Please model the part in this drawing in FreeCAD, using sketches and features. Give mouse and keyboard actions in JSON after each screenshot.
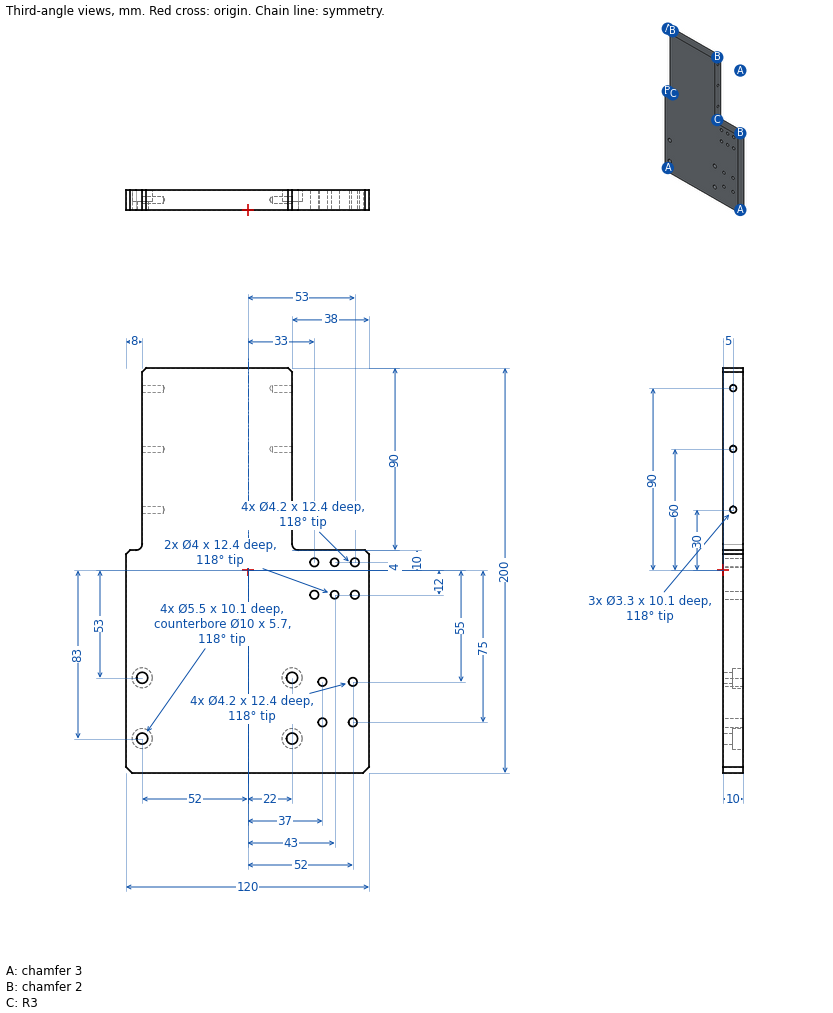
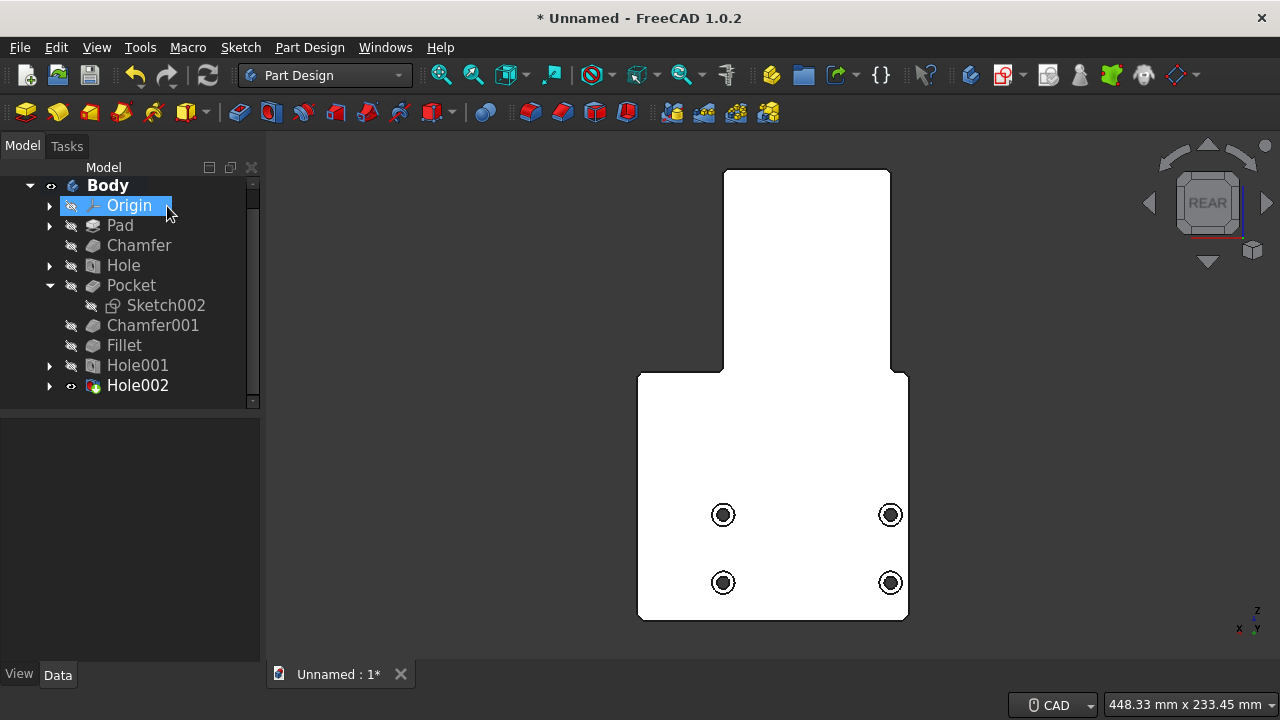
{"action": "left_click", "coordinate": [812, 459]}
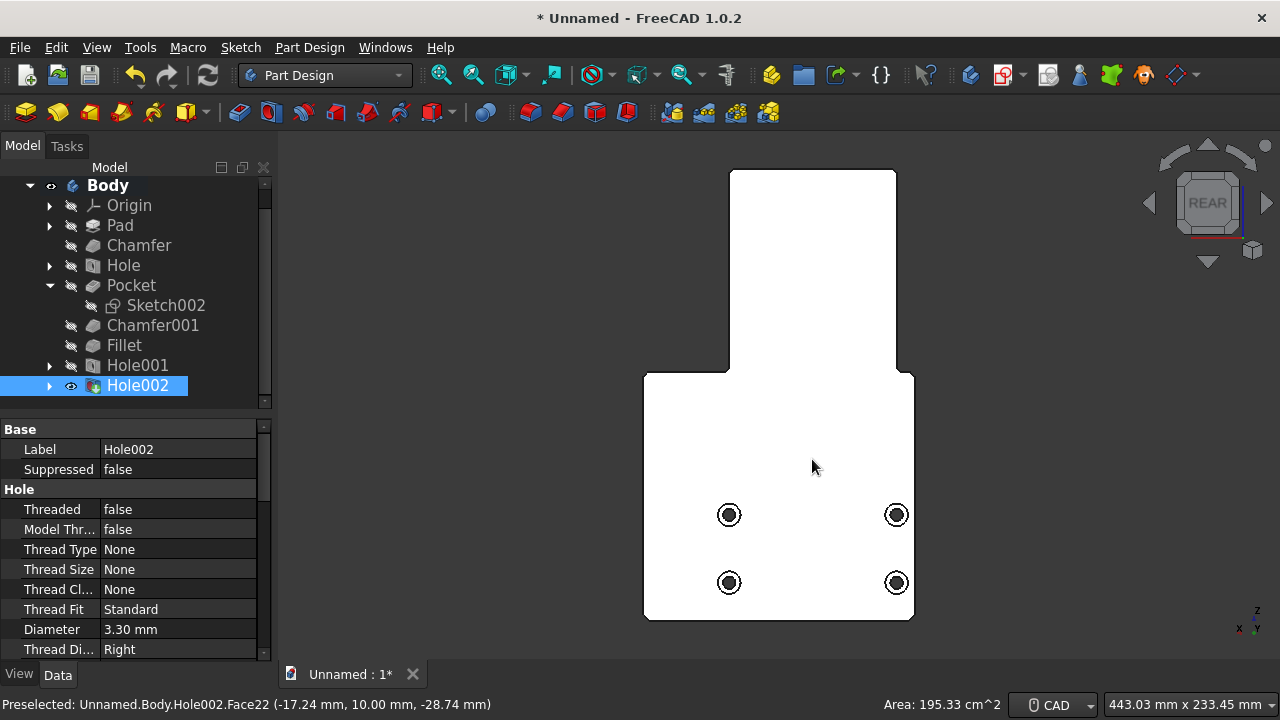
{"action": "left_click", "coordinate": [1004, 76]}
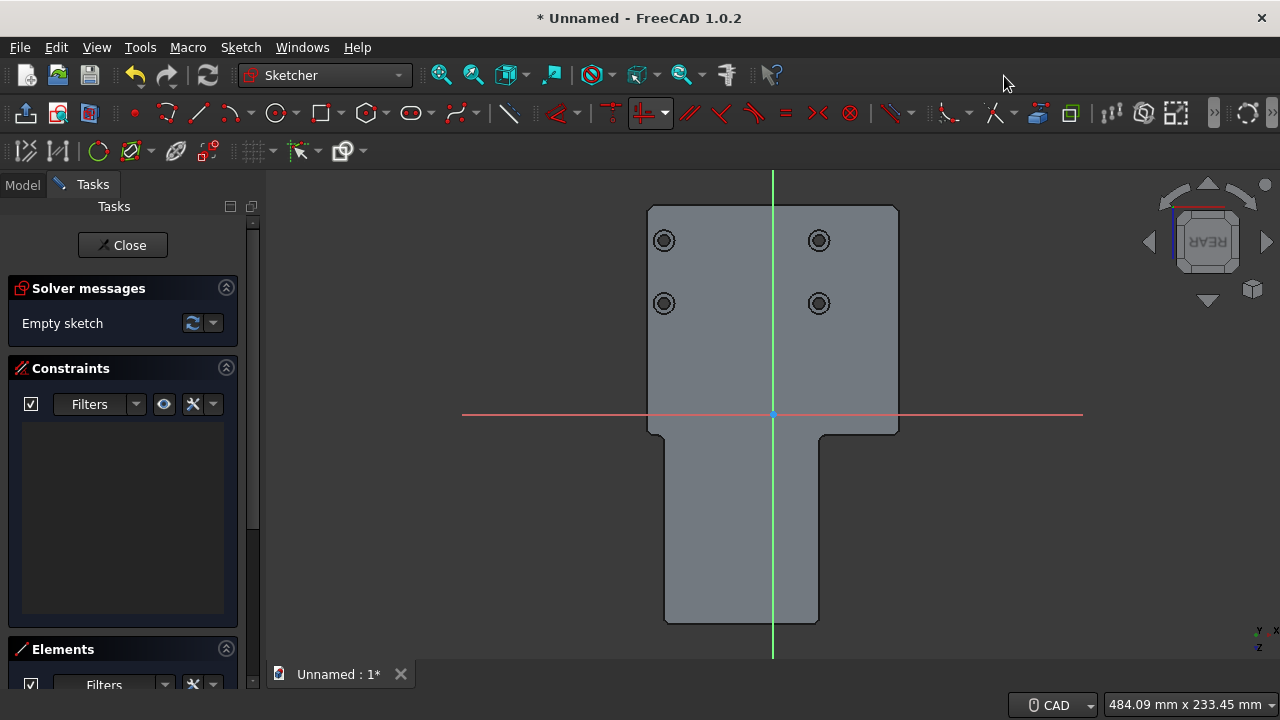
{"action": "scroll", "coordinate": [843, 404], "scroll_direction": "up", "scroll_amount": 9}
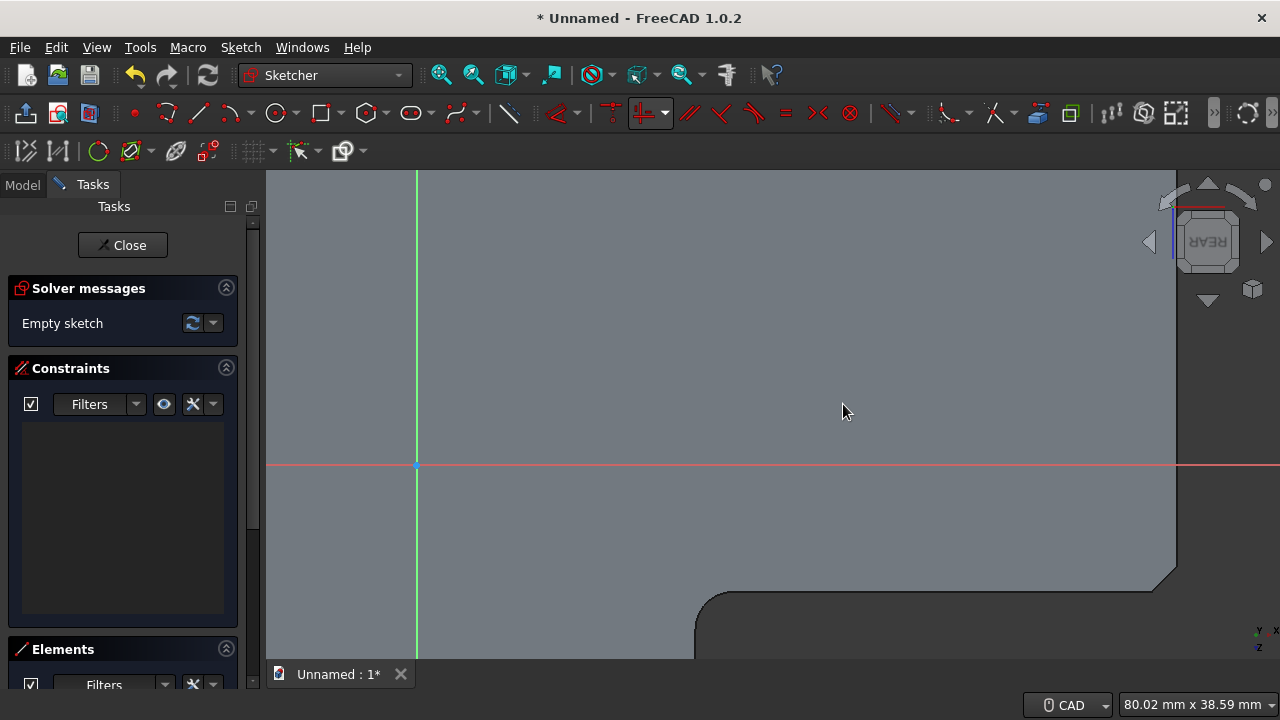
{"action": "left_click", "coordinate": [276, 114]}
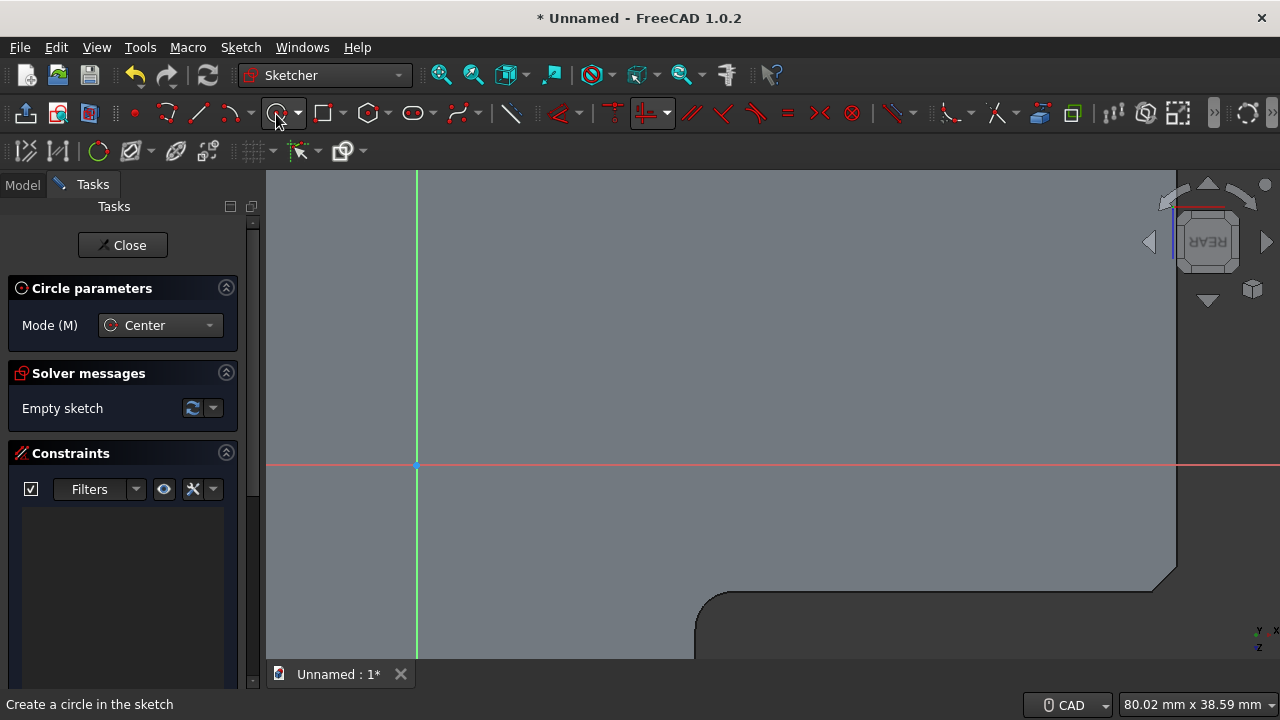
{"action": "left_click", "coordinate": [962, 313]}
{"action": "left_click", "coordinate": [979, 295]}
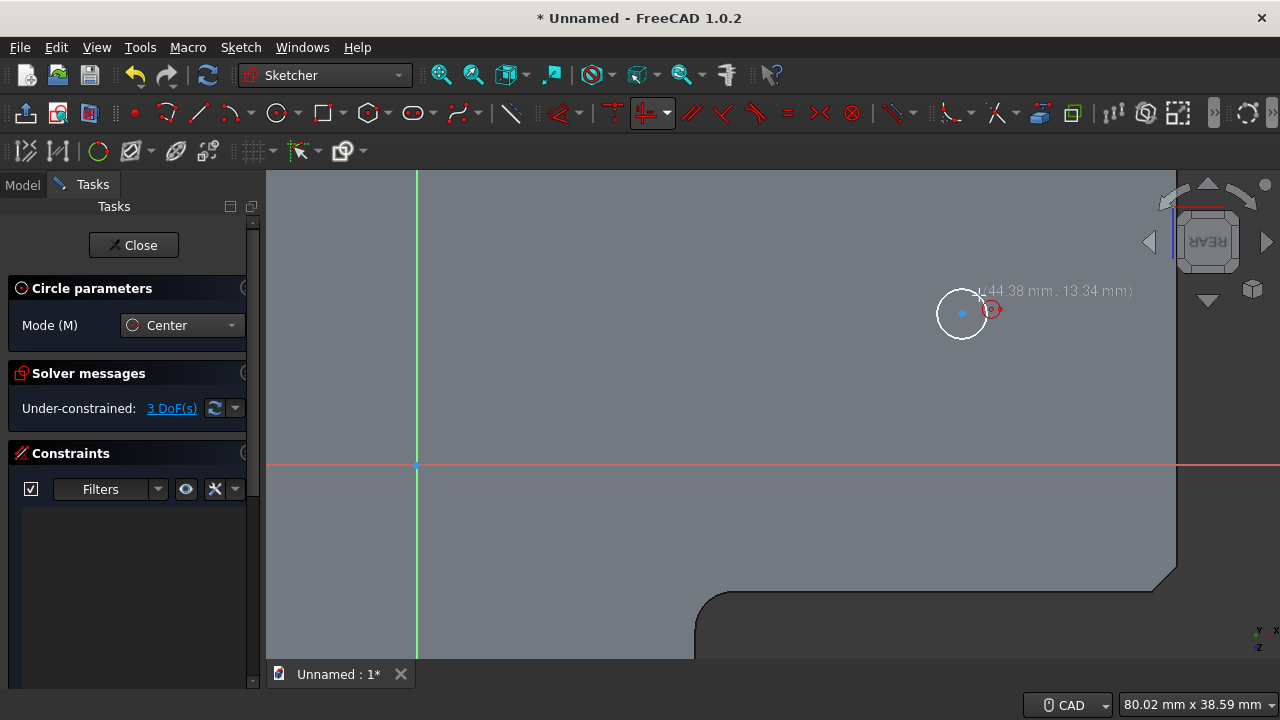
{"action": "left_click", "coordinate": [962, 516]}
{"action": "left_click", "coordinate": [979, 498]}
{"action": "key", "text": "Escape"}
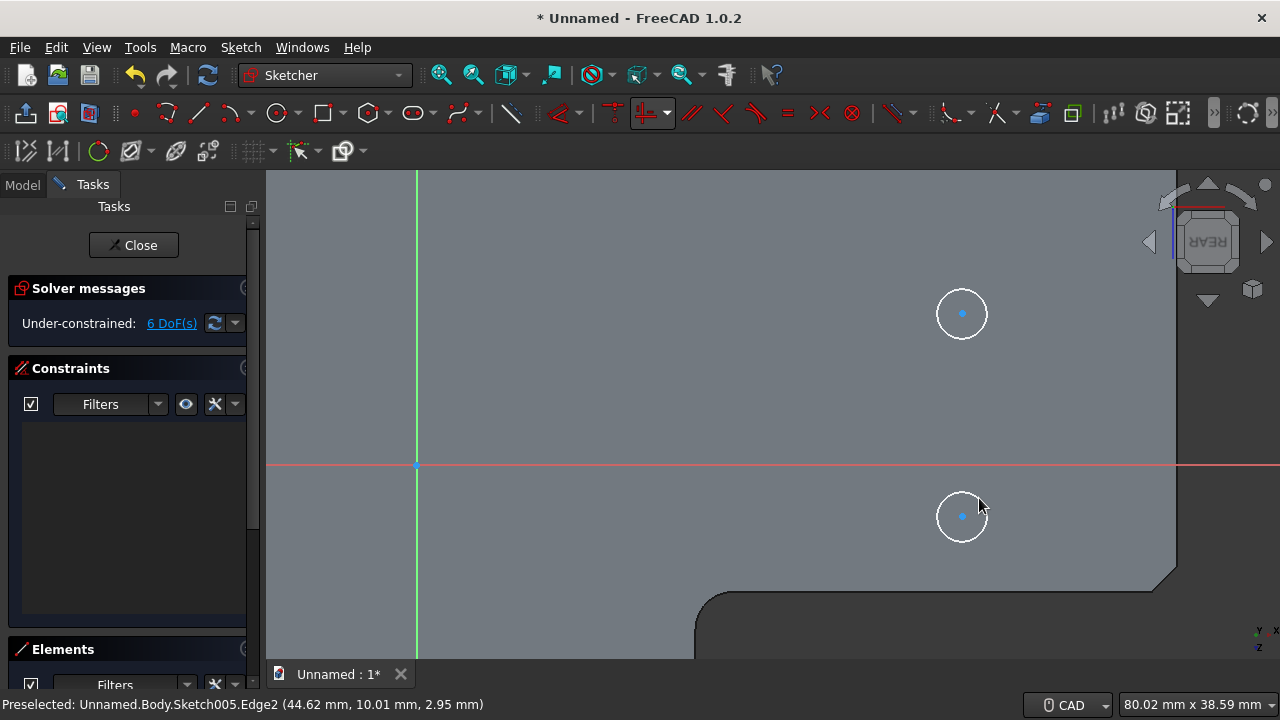
{"action": "left_click", "coordinate": [979, 296]}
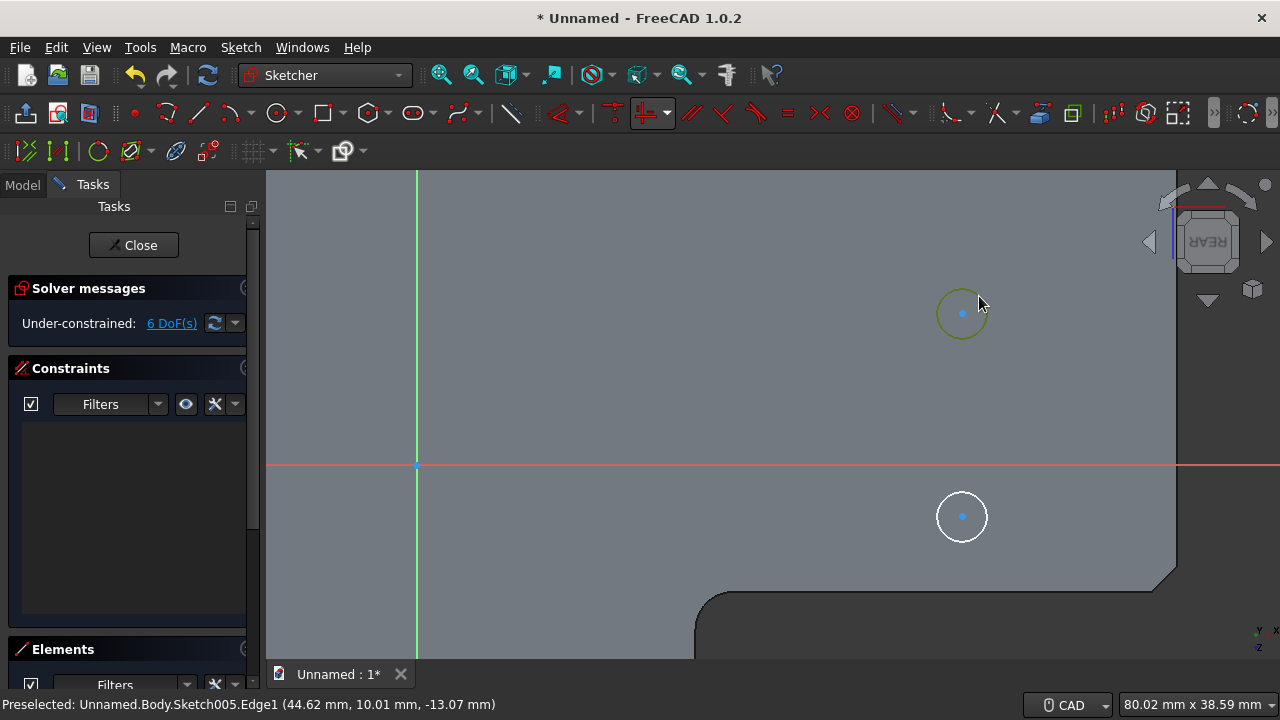
{"action": "left_click", "coordinate": [979, 499]}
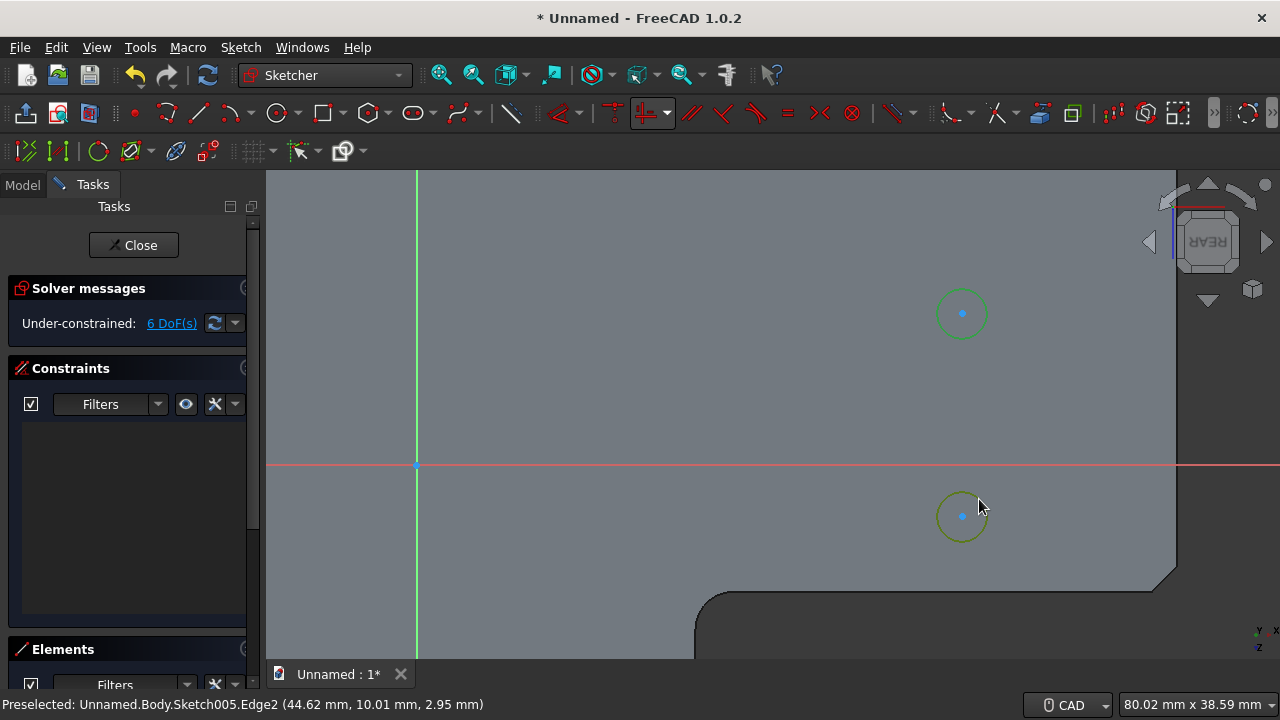
{"action": "left_click", "coordinate": [788, 114]}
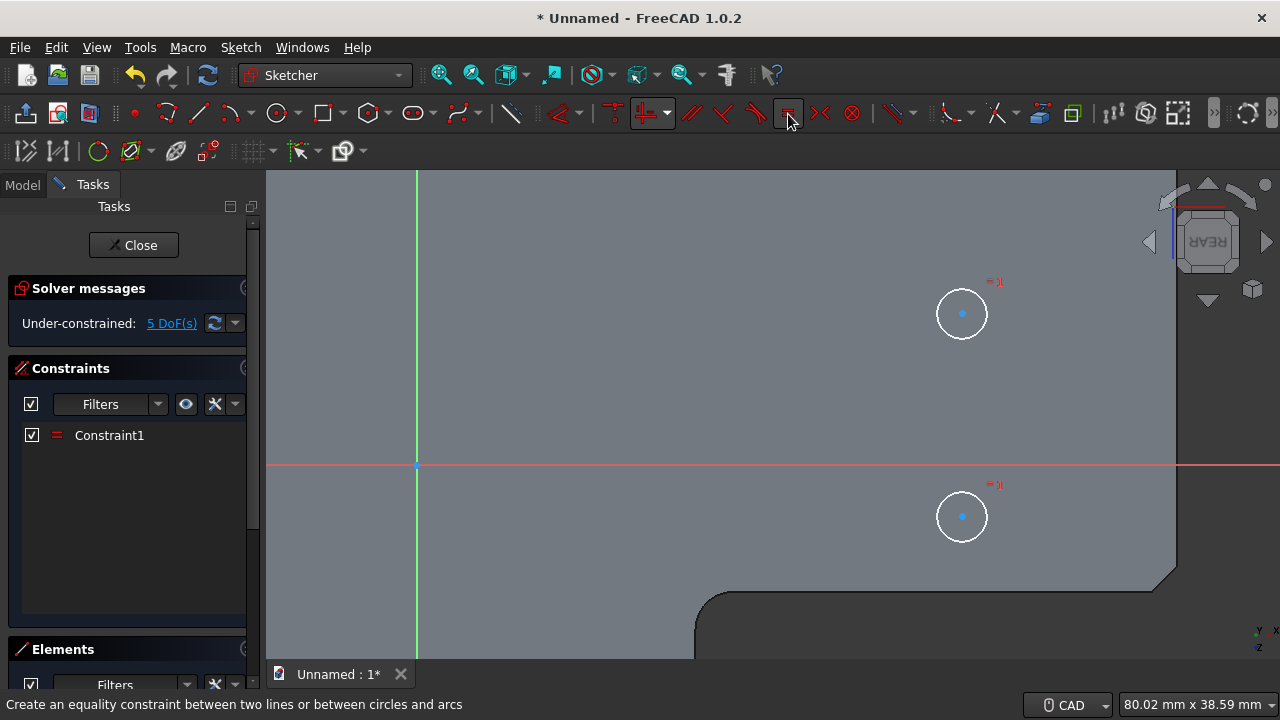
{"action": "left_click", "coordinate": [962, 314]}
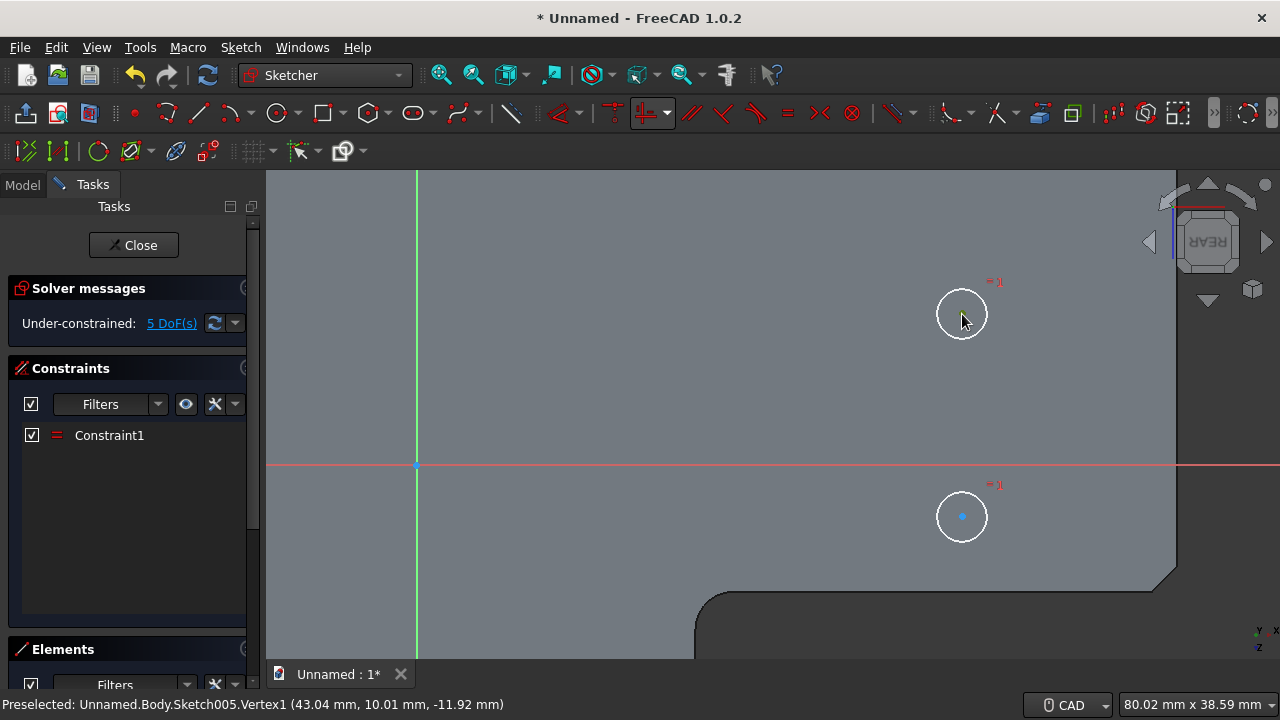
{"action": "left_click", "coordinate": [962, 517]}